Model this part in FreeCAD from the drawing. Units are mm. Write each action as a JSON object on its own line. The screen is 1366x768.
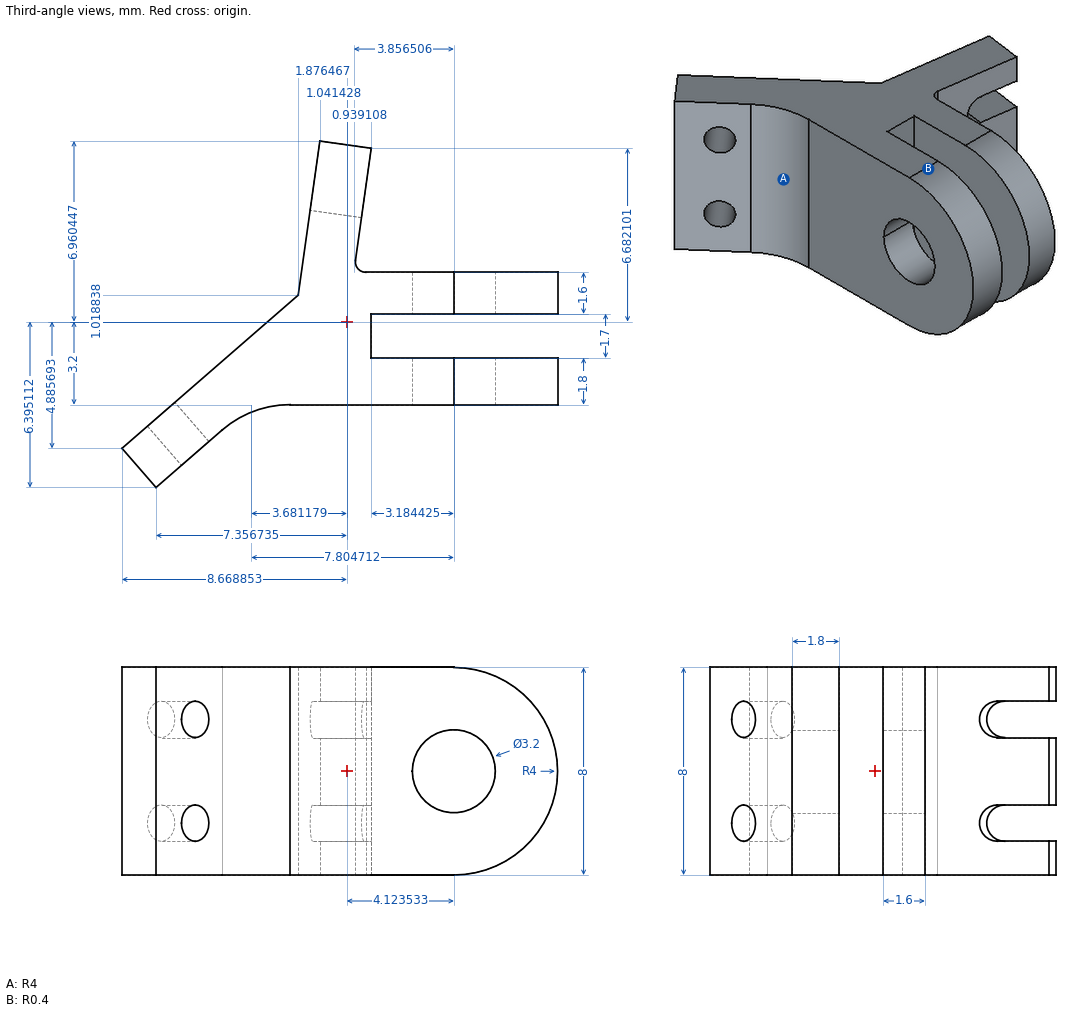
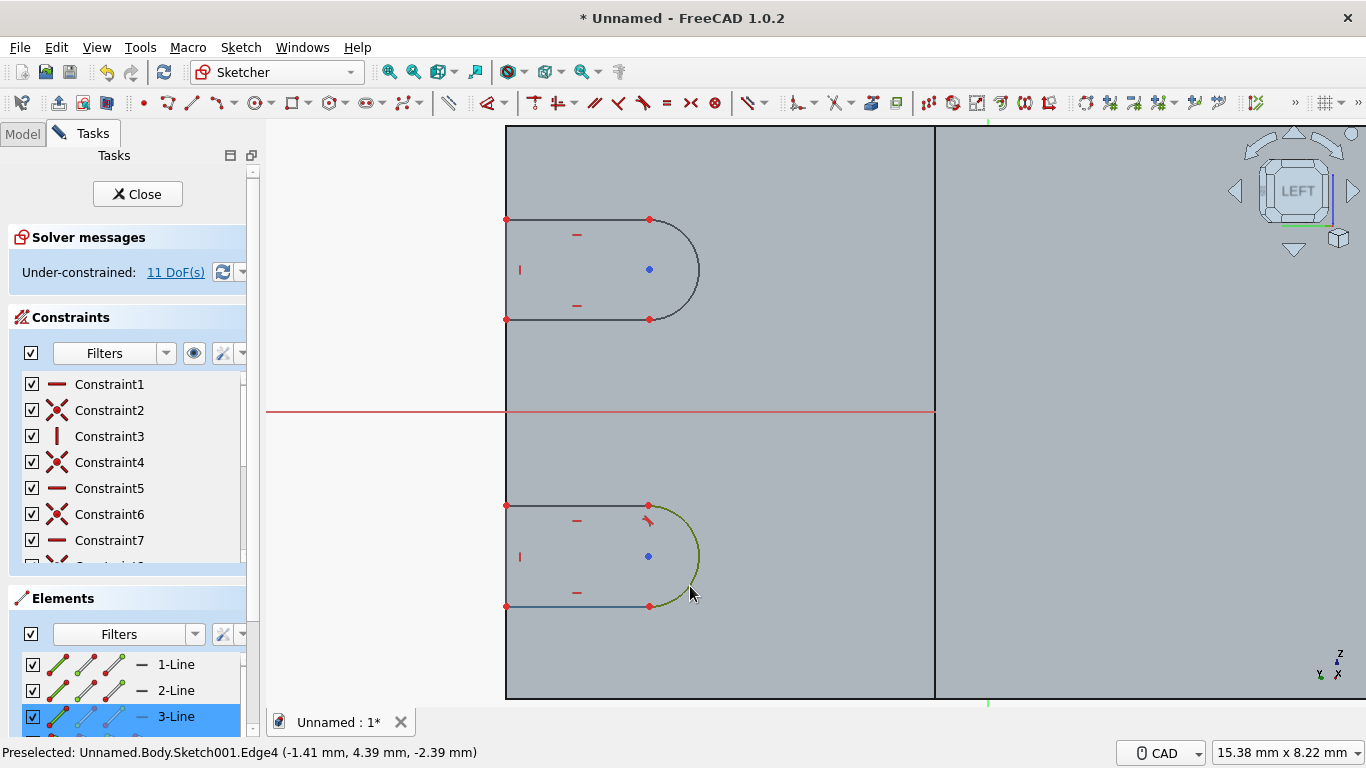
{"action": "left_click", "coordinate": [644, 104]}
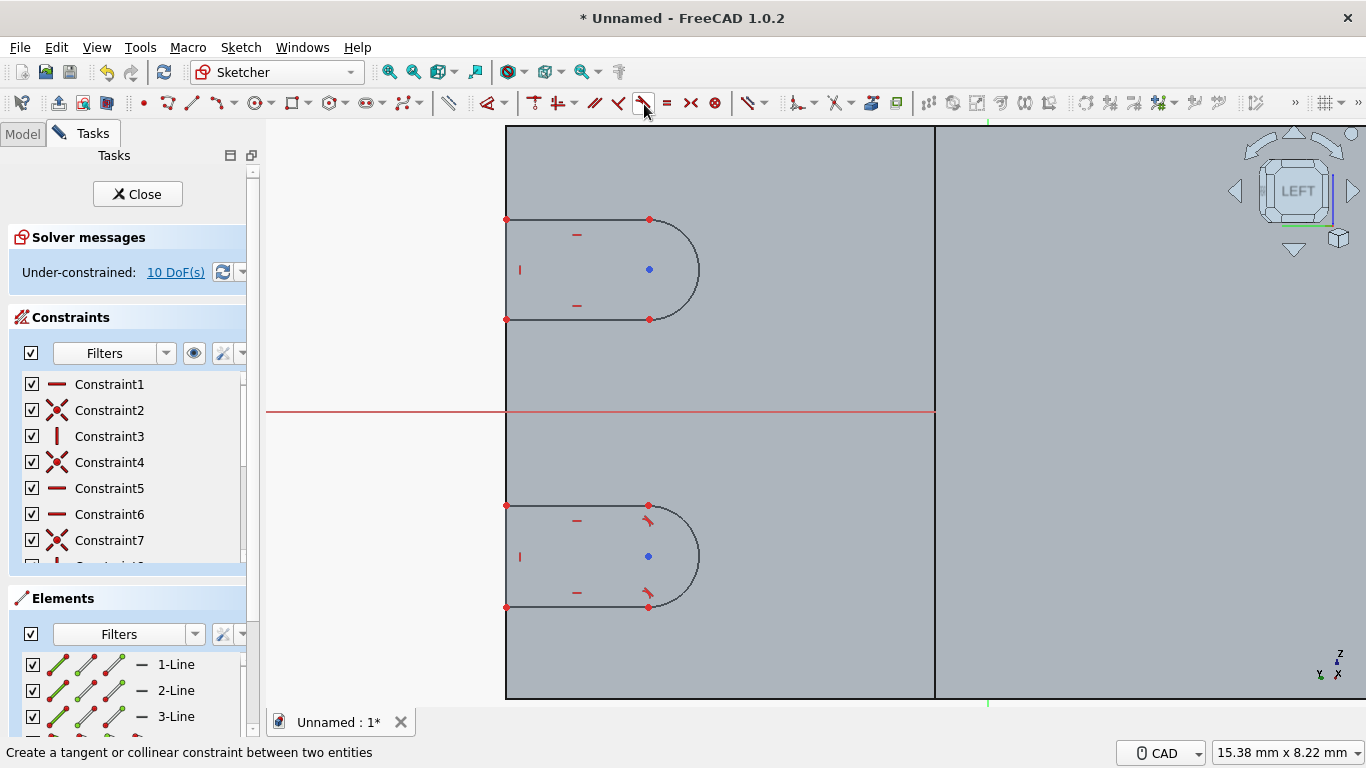
{"action": "left_click", "coordinate": [606, 220]}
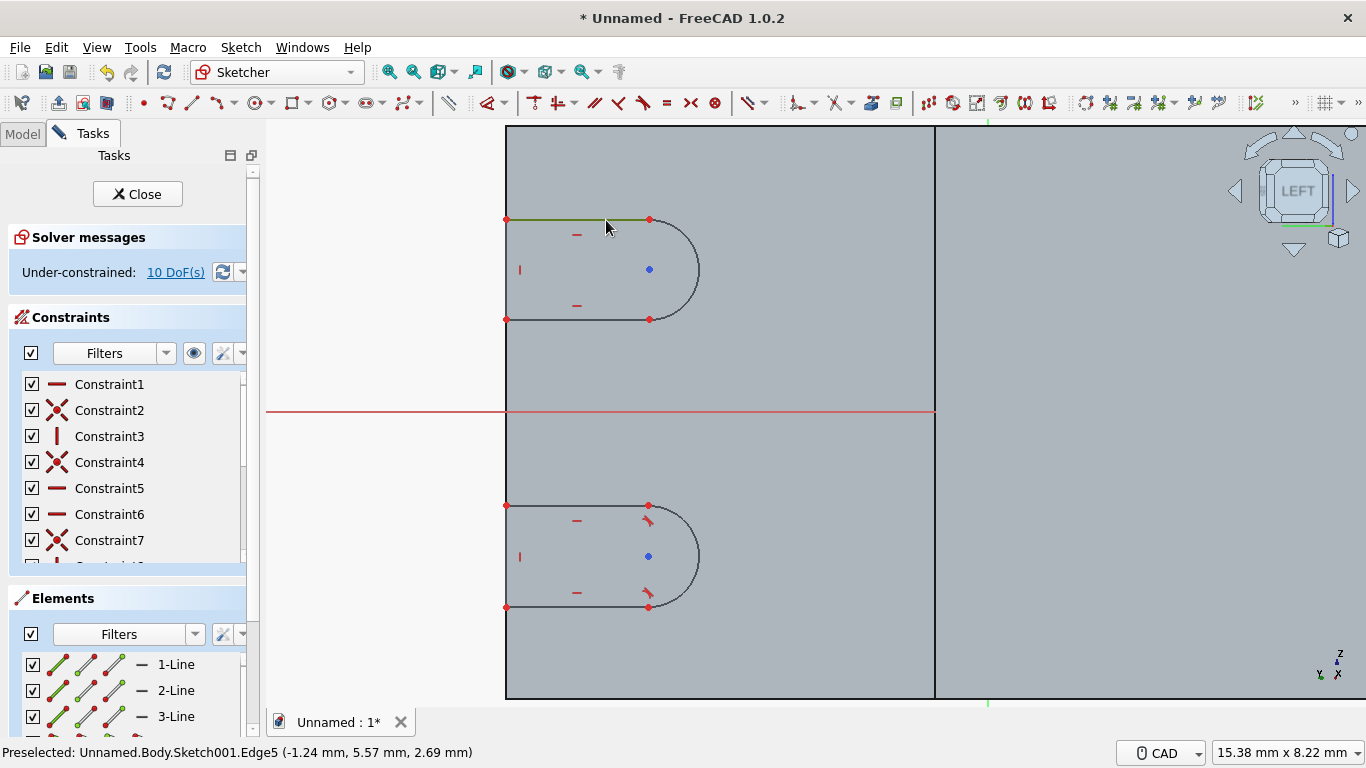
{"action": "left_click", "coordinate": [689, 299]}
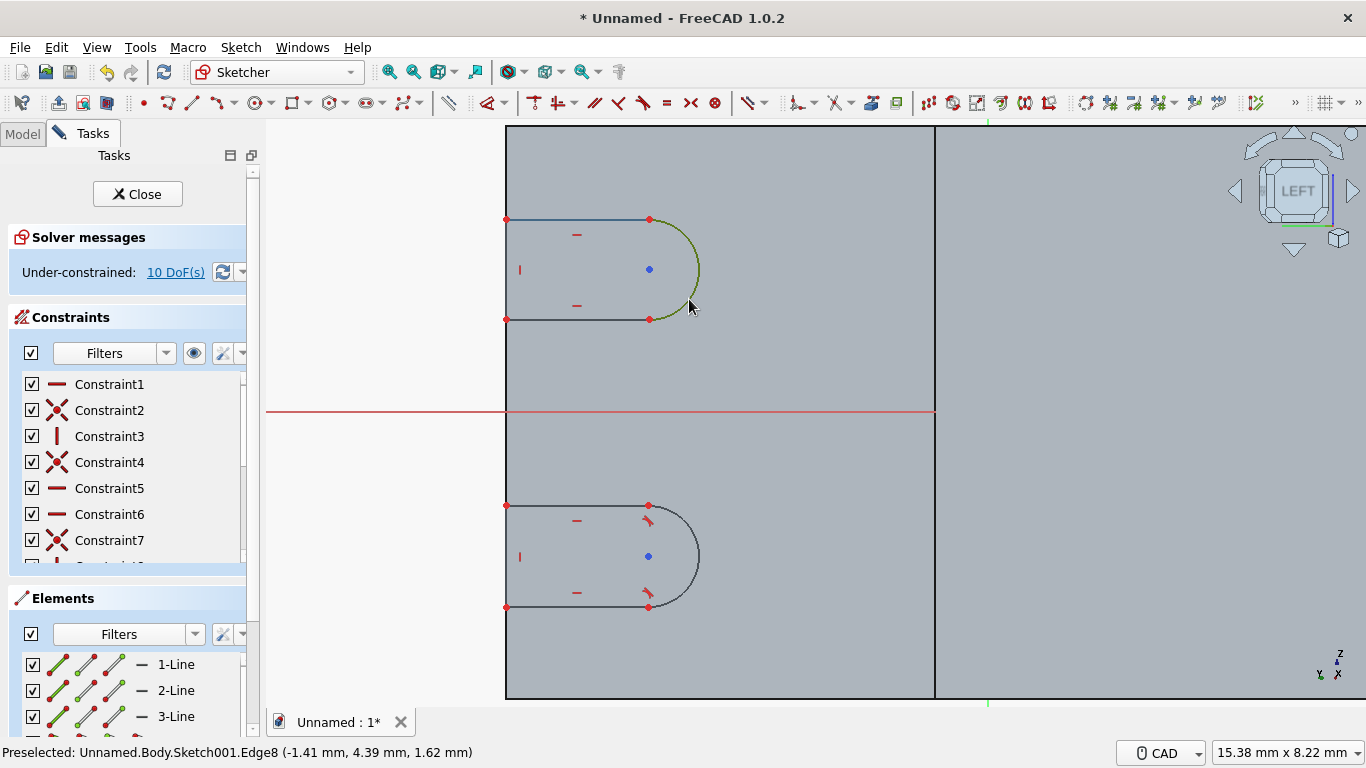
{"action": "left_click", "coordinate": [644, 104]}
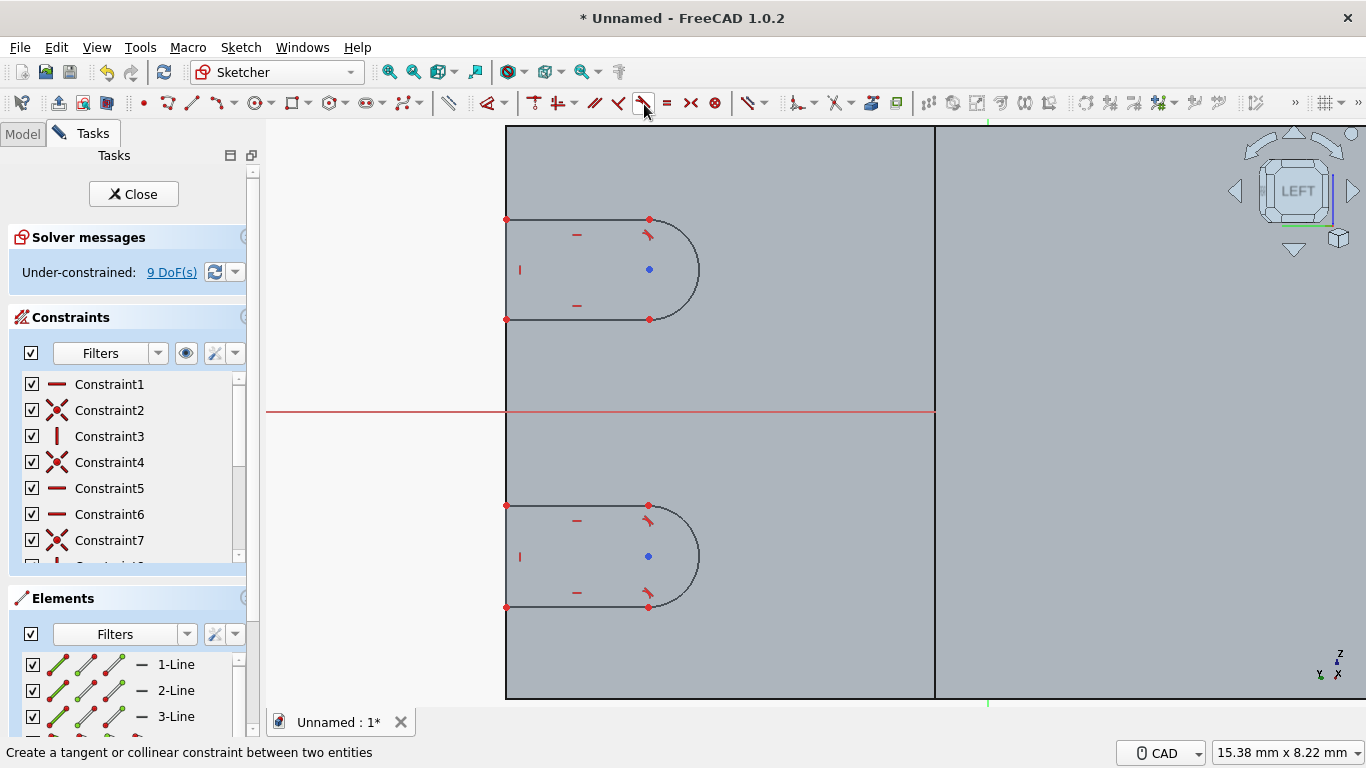
{"action": "left_click", "coordinate": [549, 320]}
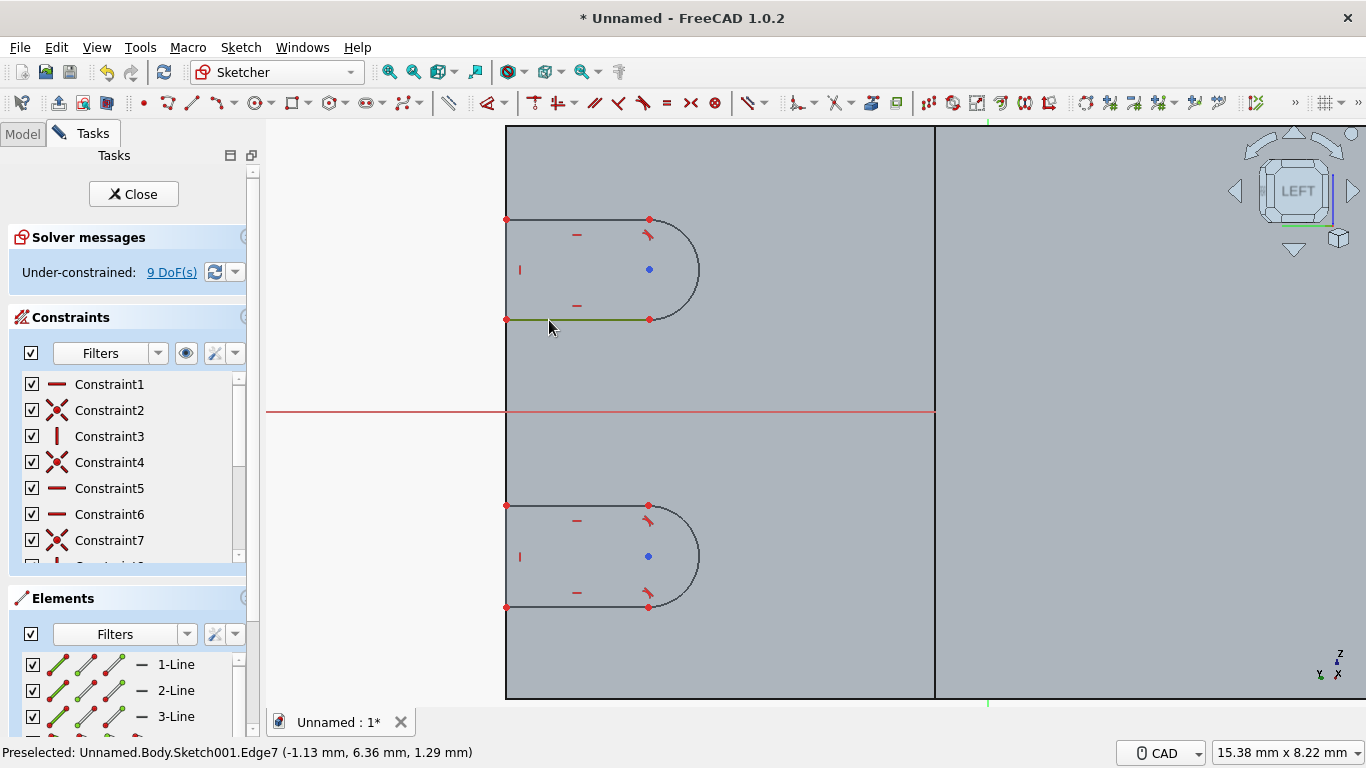
{"action": "left_click", "coordinate": [689, 299]}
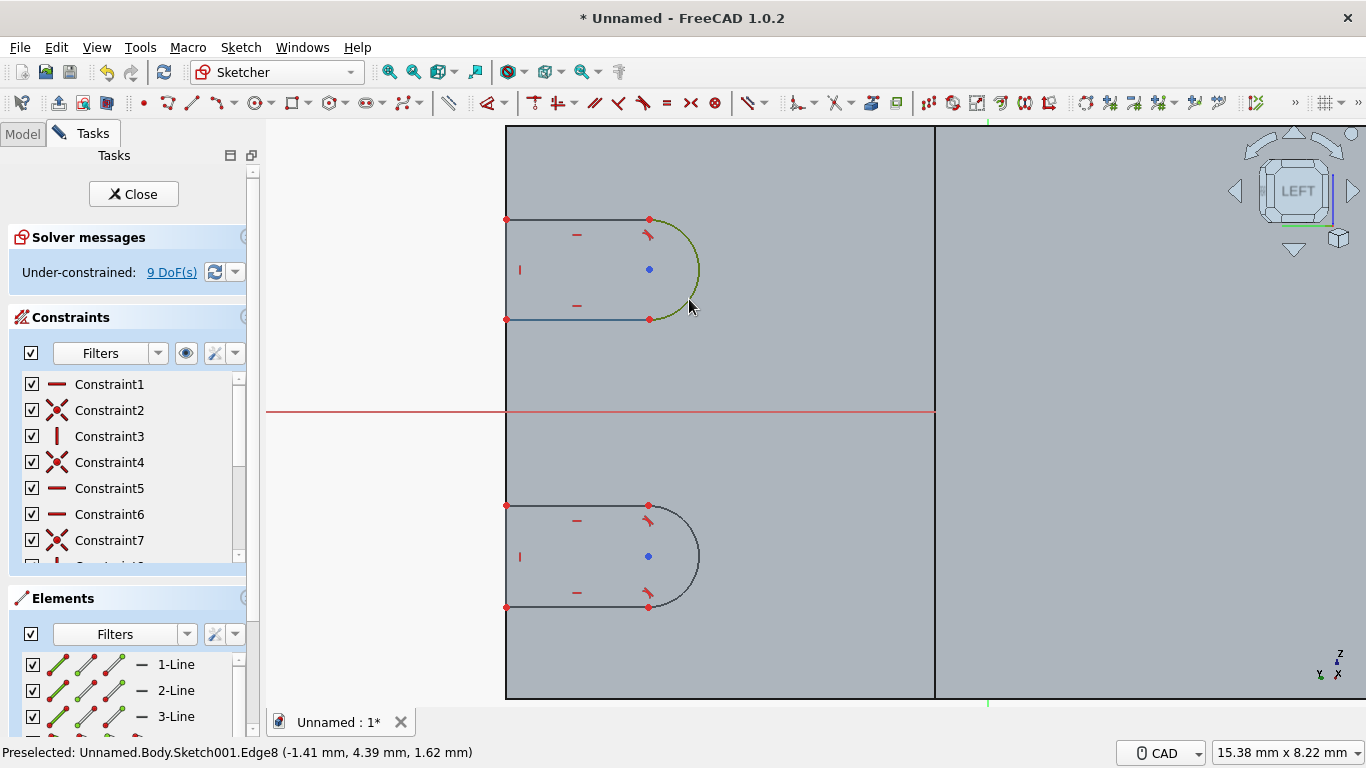
{"action": "left_click", "coordinate": [644, 104]}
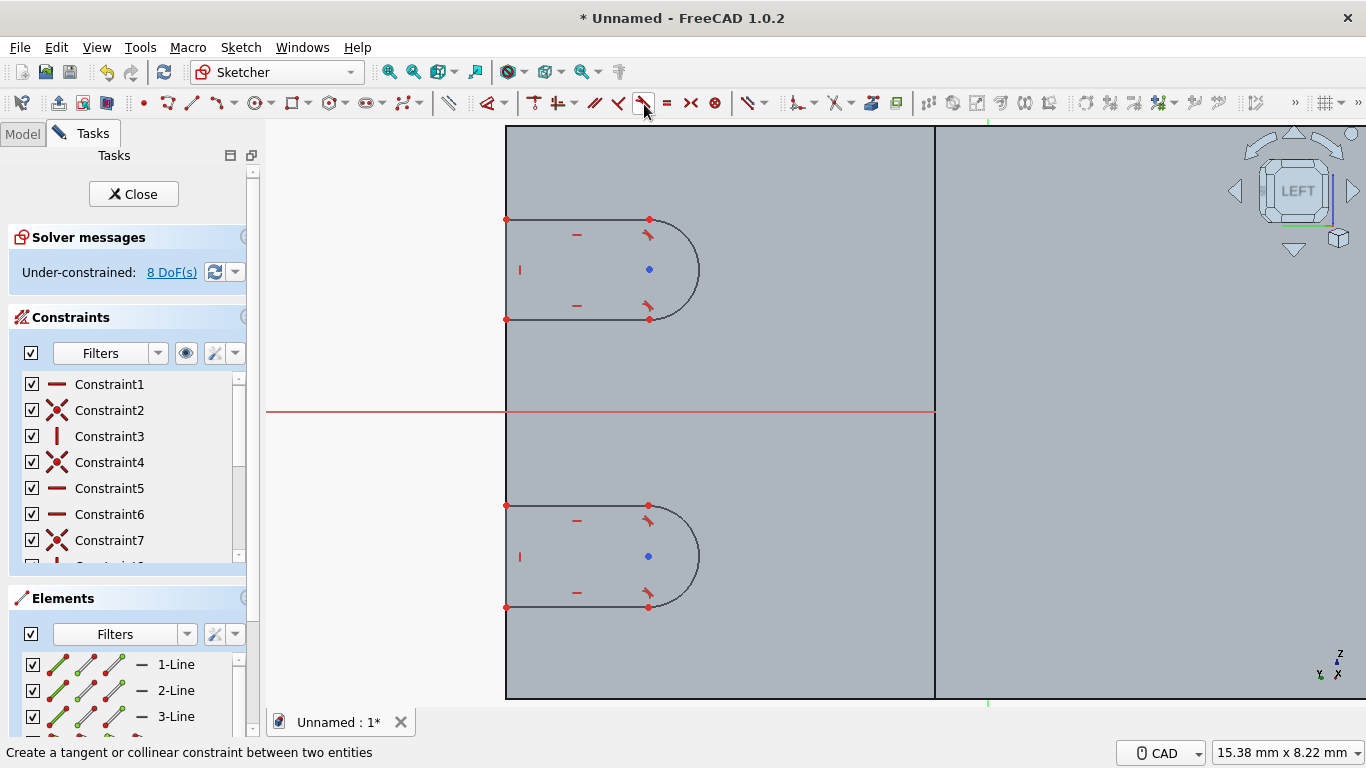
{"action": "left_click", "coordinate": [689, 586]}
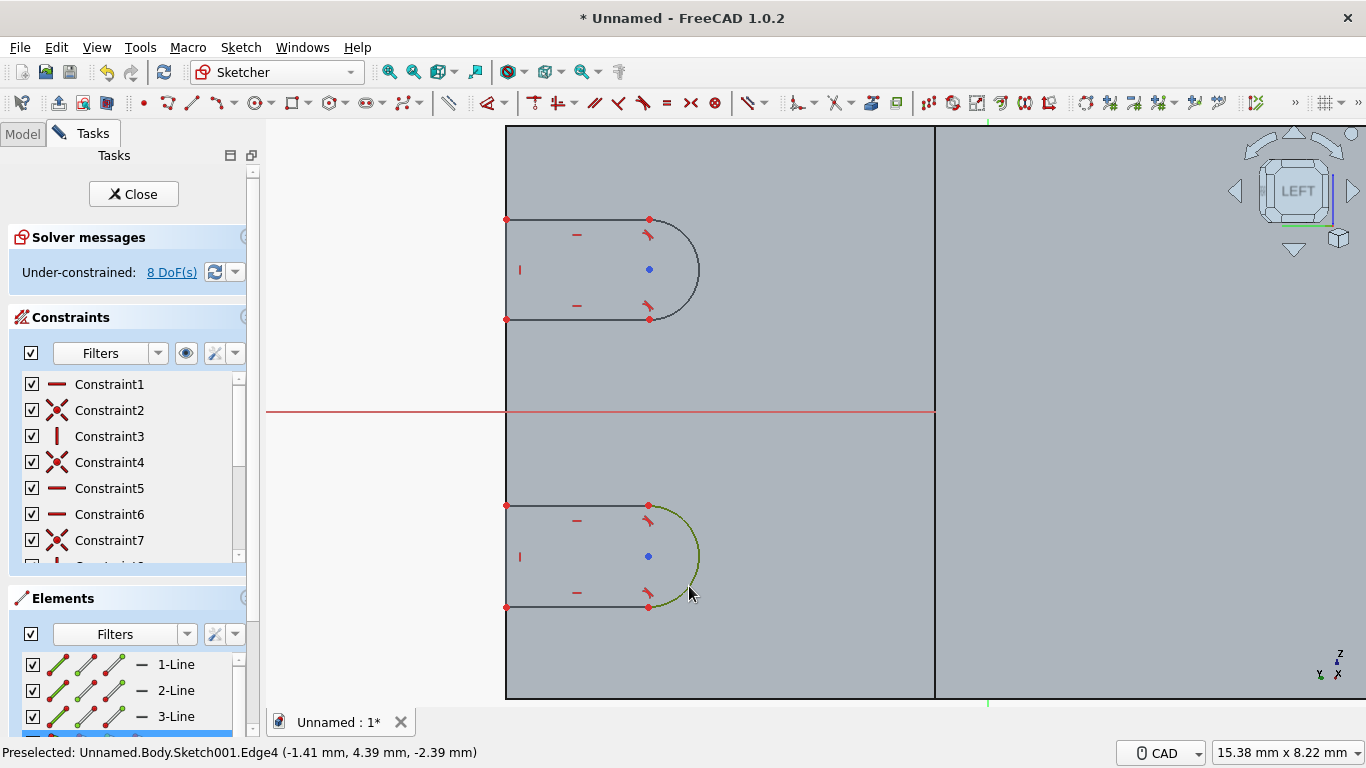
{"action": "left_click", "coordinate": [689, 299]}